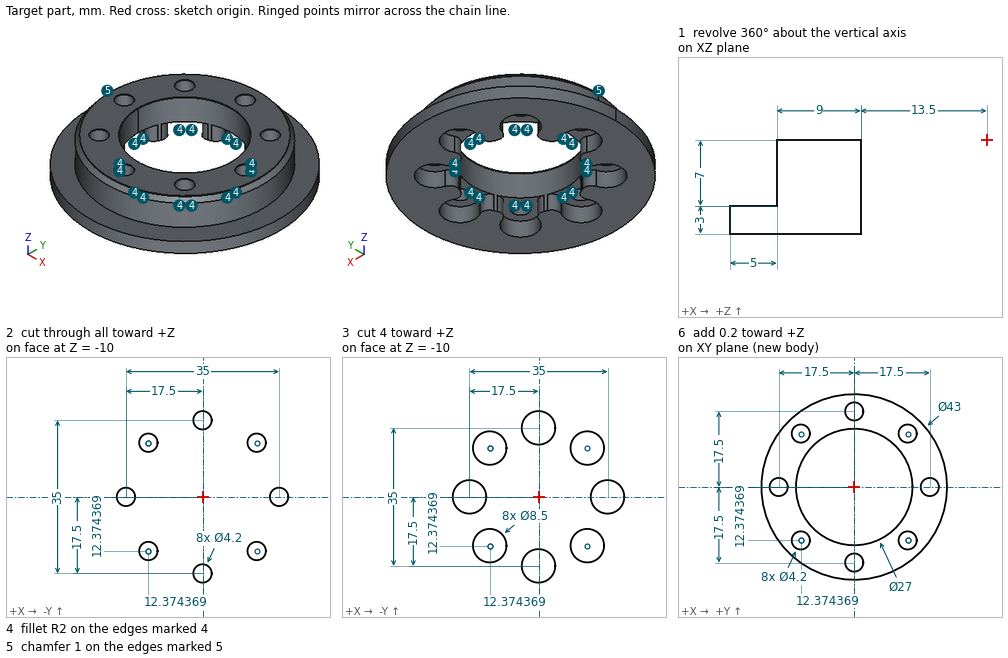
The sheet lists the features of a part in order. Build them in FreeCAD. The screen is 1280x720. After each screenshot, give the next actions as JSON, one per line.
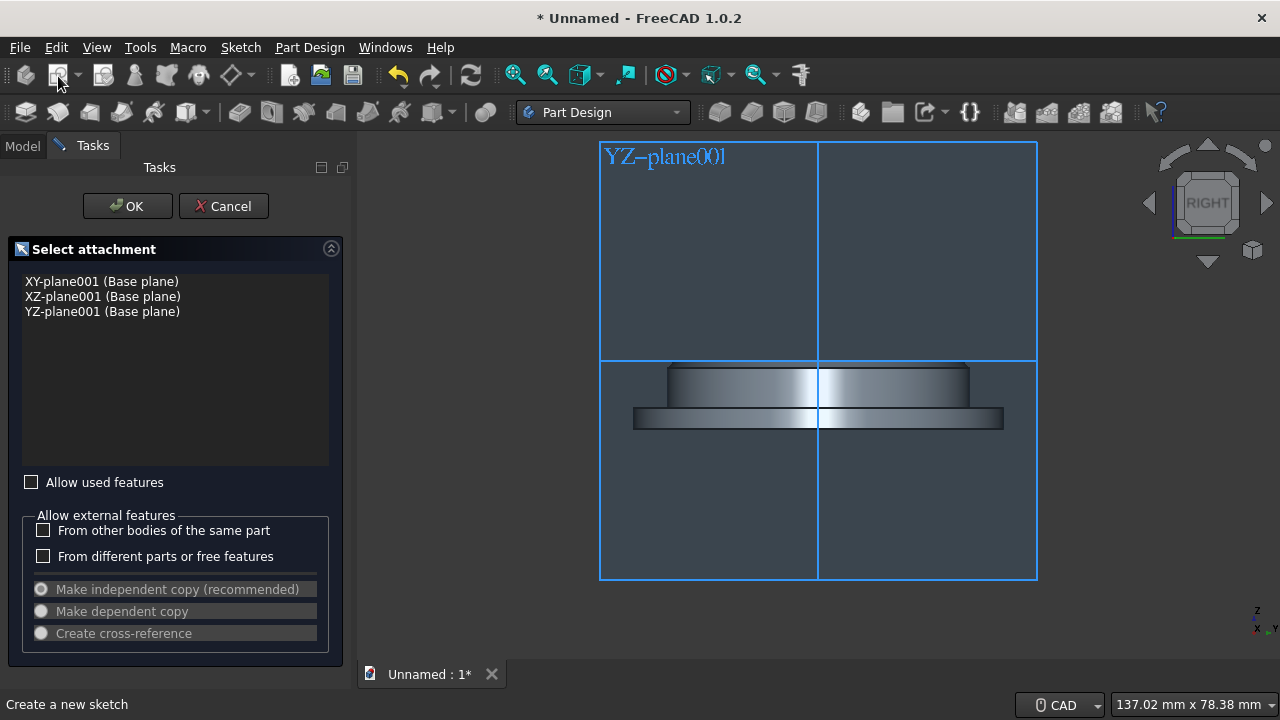
{"action": "left_click", "coordinate": [82, 282]}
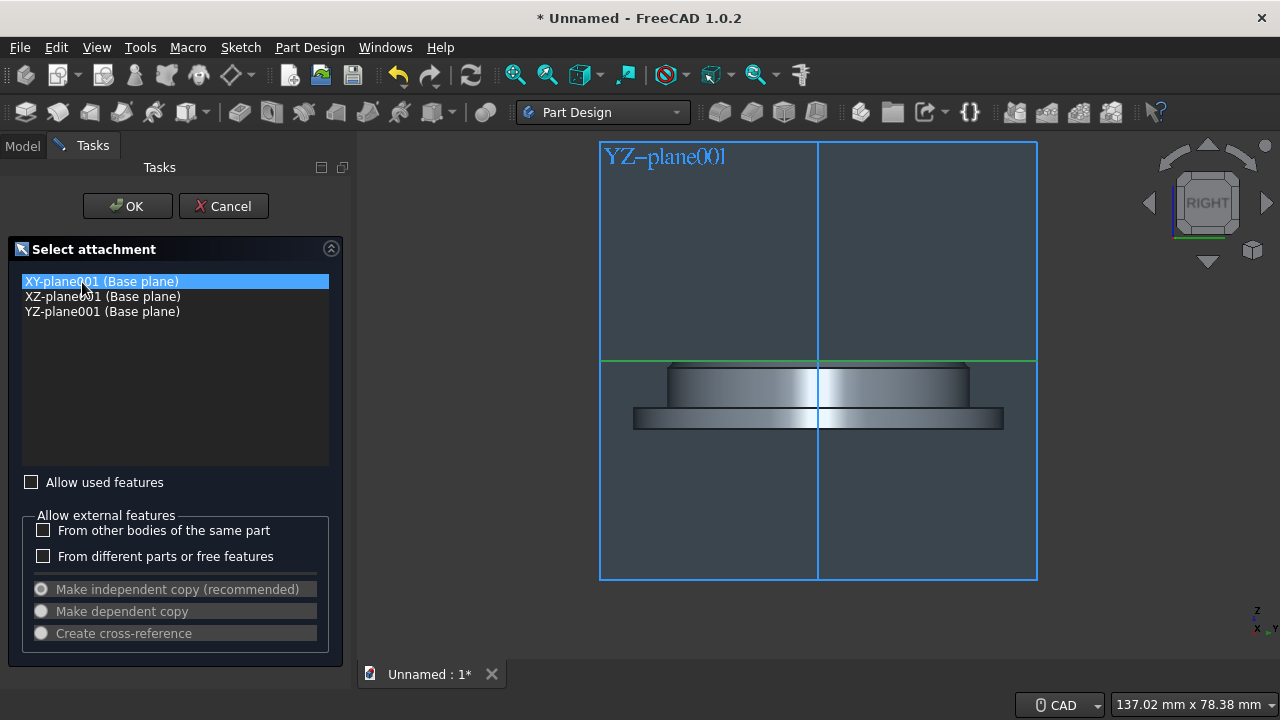
{"action": "left_click", "coordinate": [128, 206]}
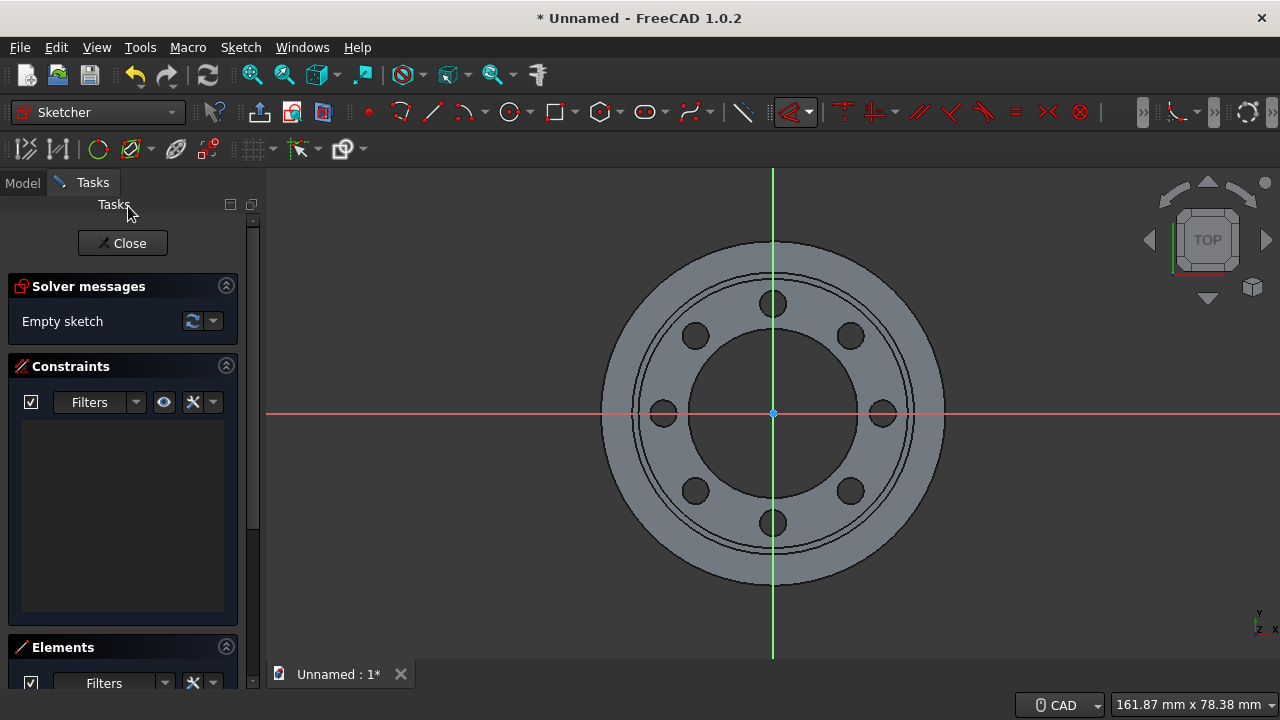
{"action": "left_click", "coordinate": [510, 112]}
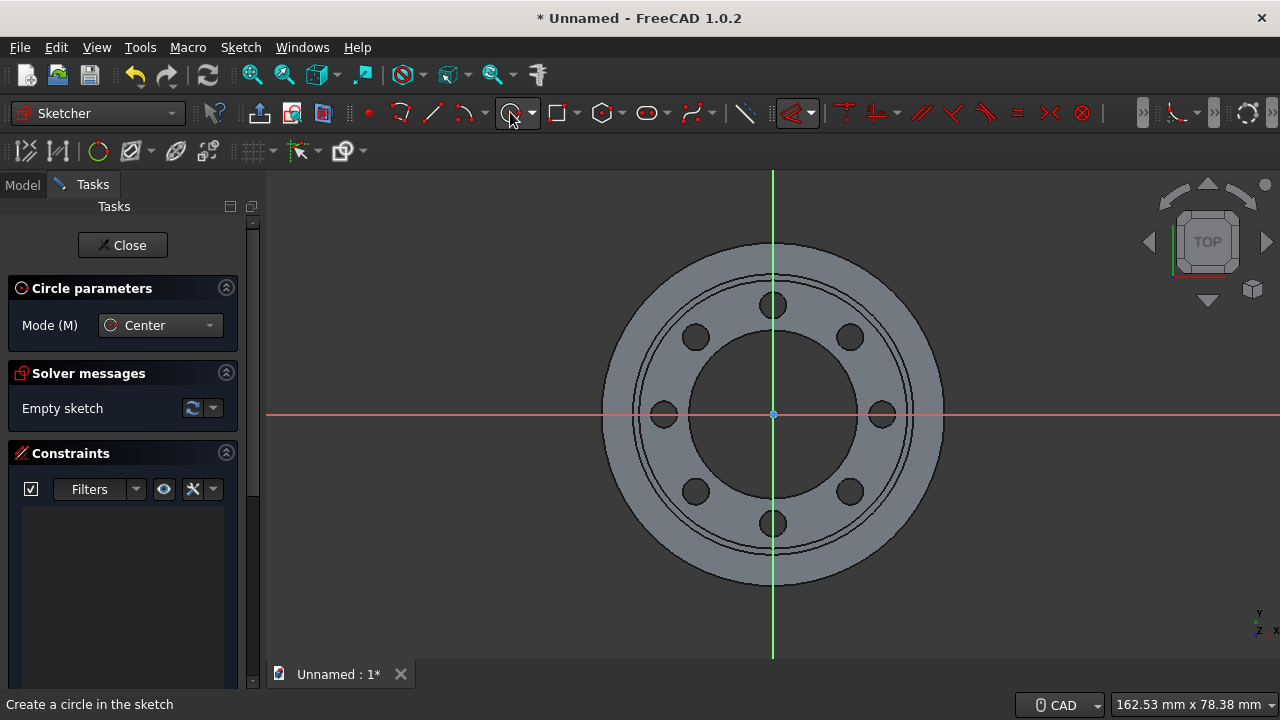
{"action": "left_click", "coordinate": [773, 415]}
{"action": "mouse_move", "coordinate": [868, 320]}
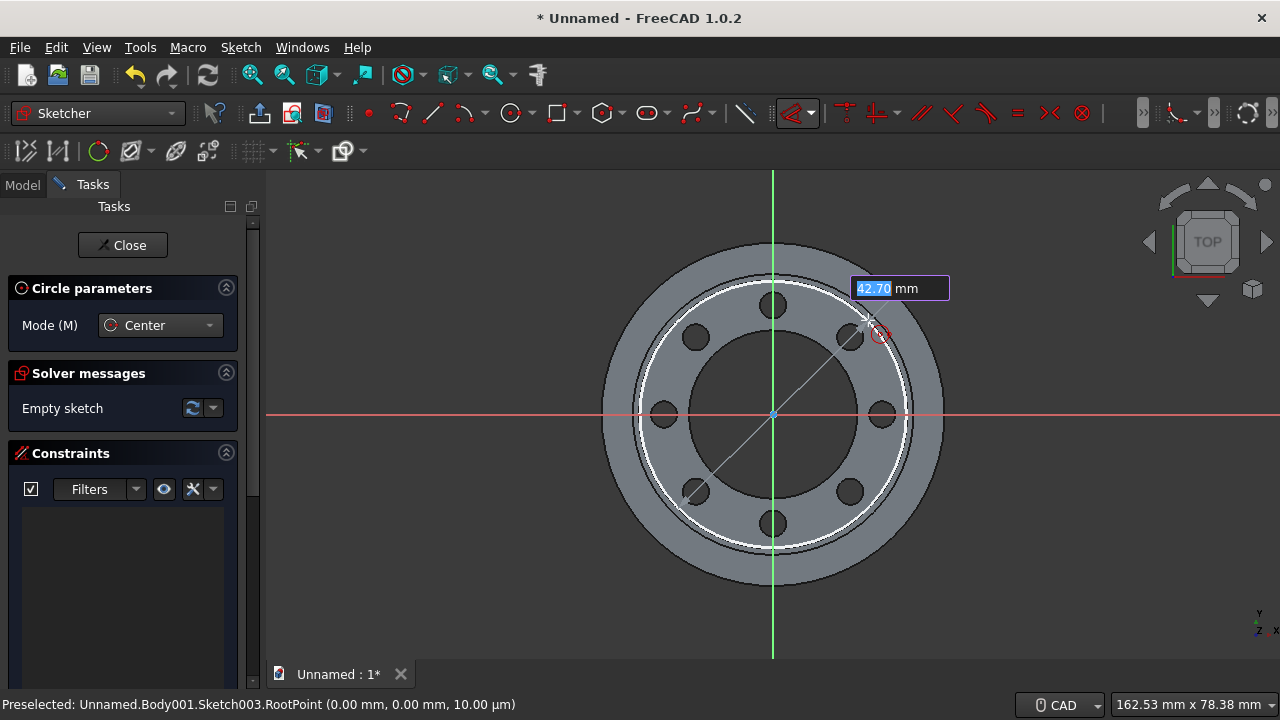
{"action": "type", "text": "43"}
{"action": "key", "text": "Return"}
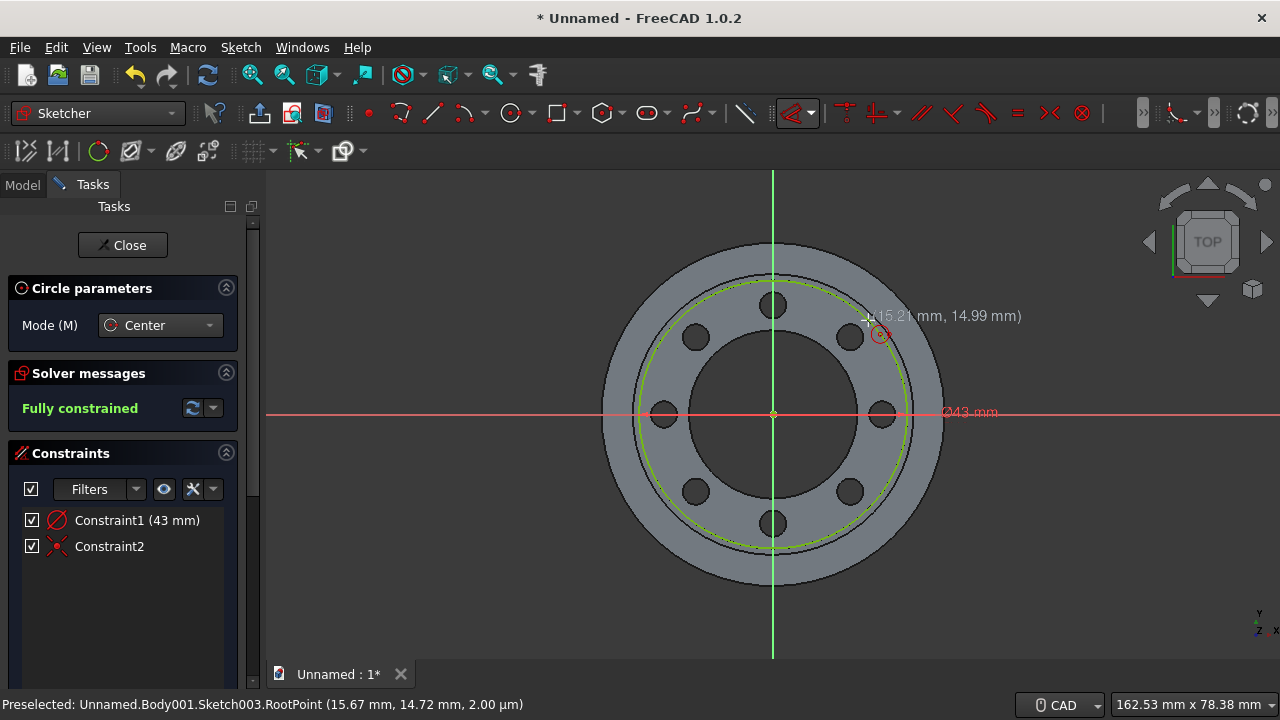
{"action": "scroll", "coordinate": [696, 492], "scroll_direction": "up", "scroll_amount": 3}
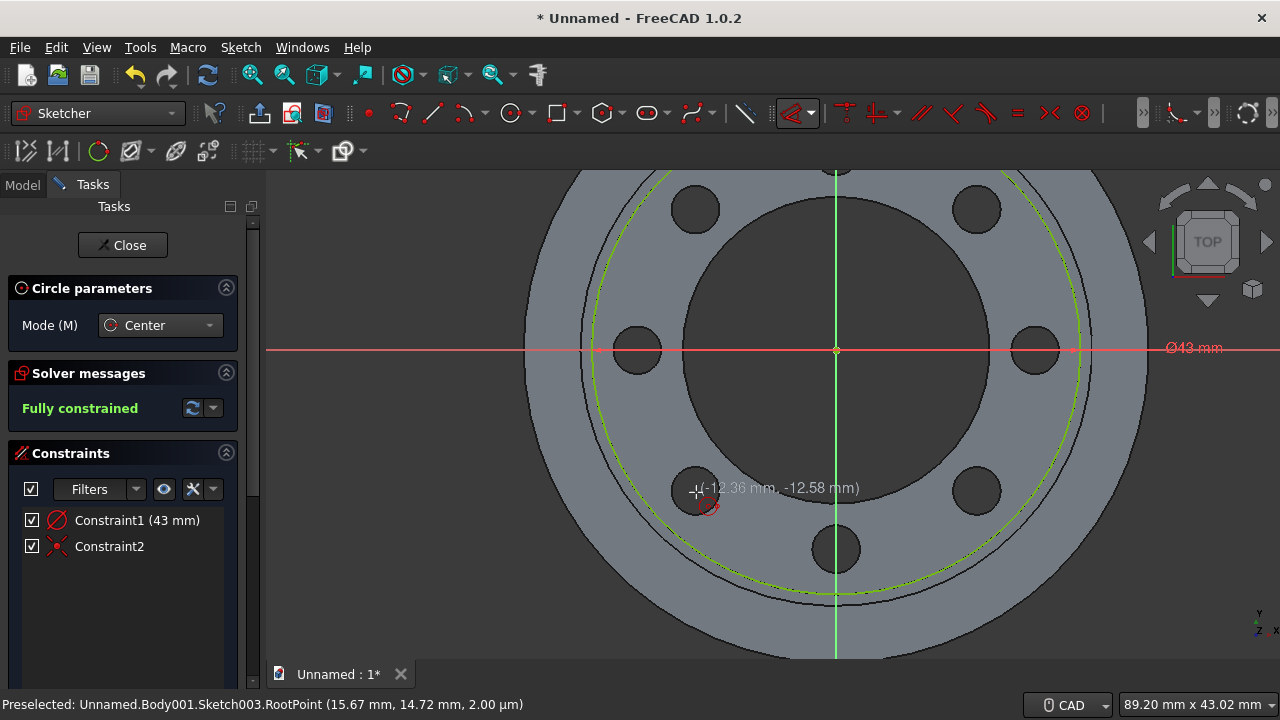
{"action": "left_click", "coordinate": [696, 491]}
{"action": "mouse_move", "coordinate": [712, 474]}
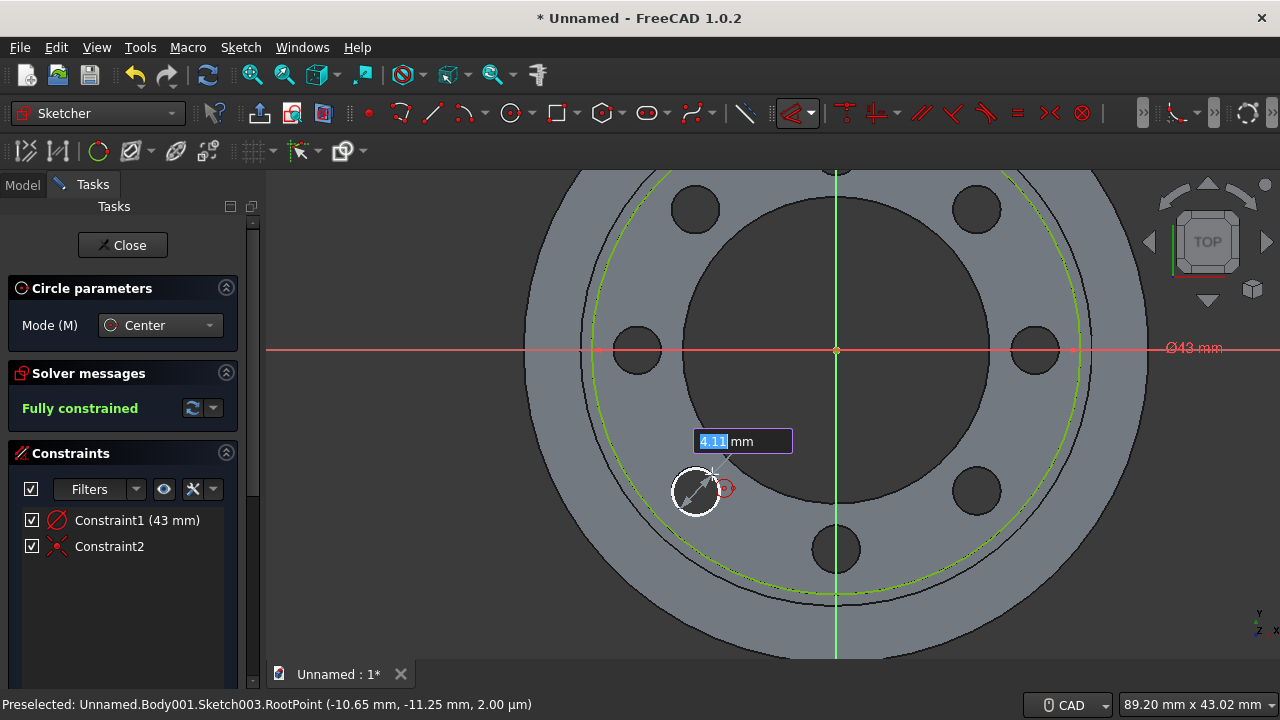
{"action": "type", "text": "4.2"}
{"action": "key", "text": "Return"}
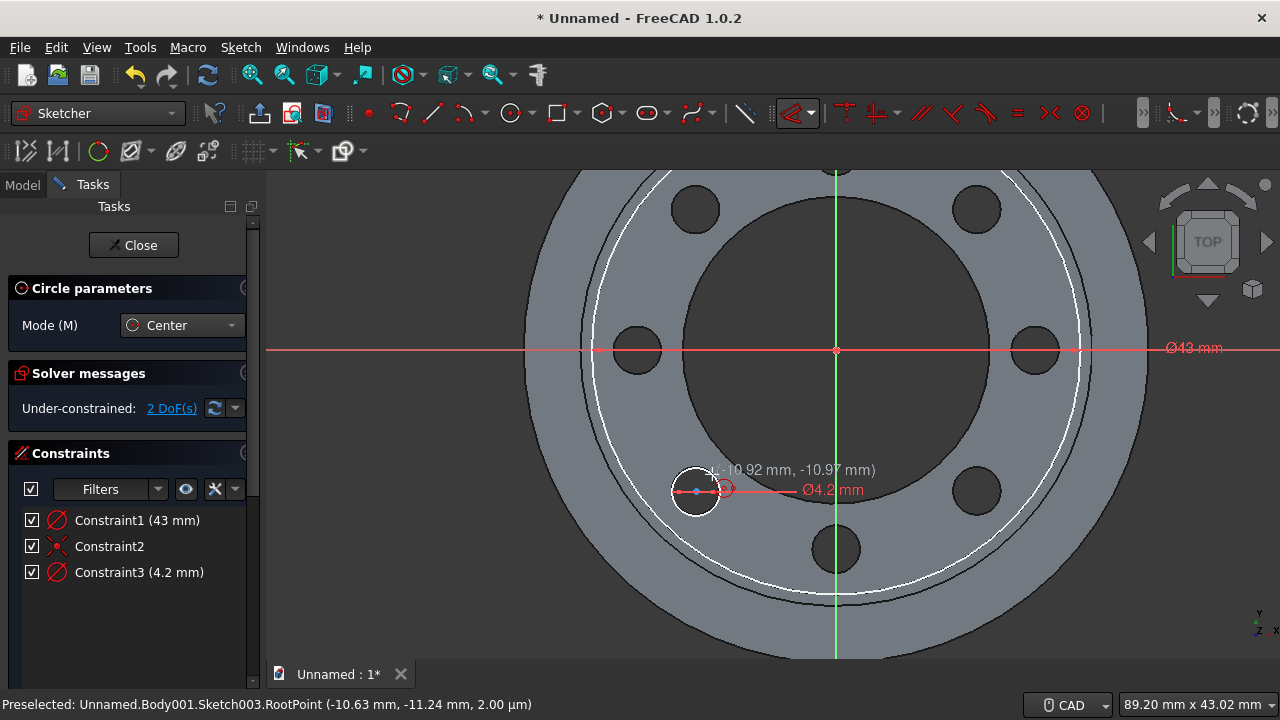
{"action": "left_click", "coordinate": [836, 549]}
{"action": "mouse_move", "coordinate": [853, 532]}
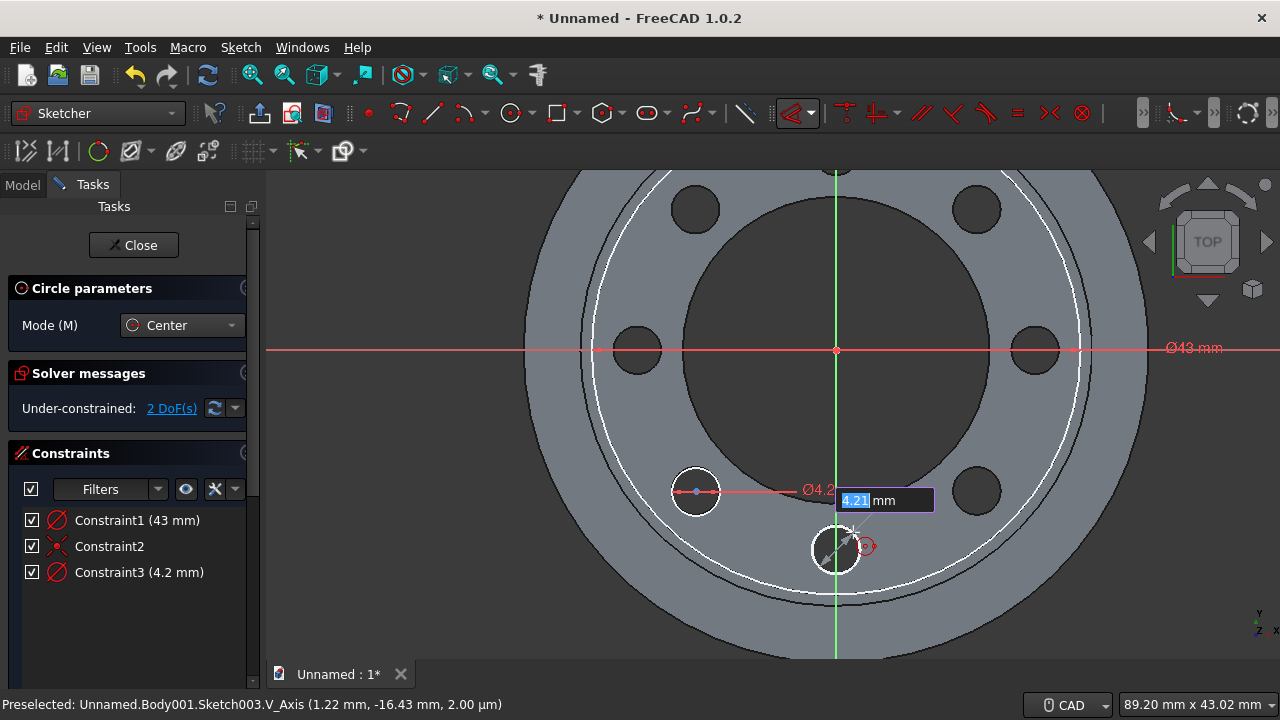
{"action": "type", "text": "4.2"}
{"action": "key", "text": "Return"}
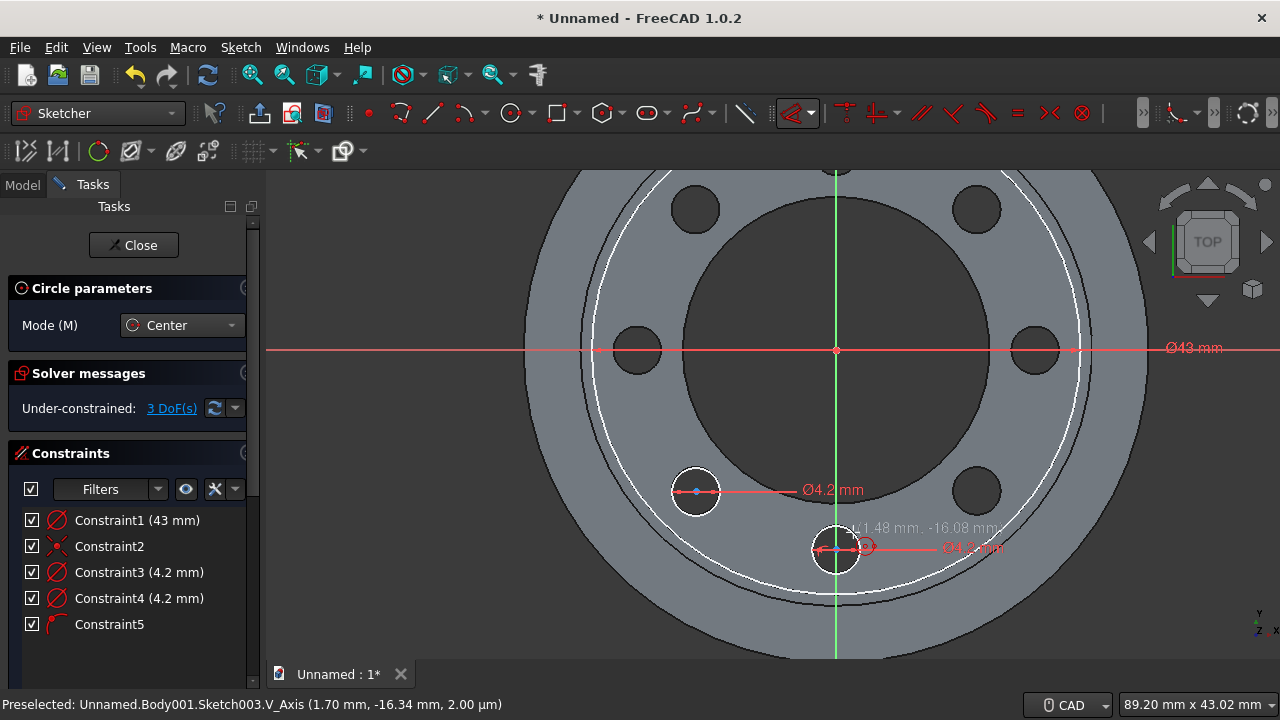
{"action": "left_click", "coordinate": [977, 491]}
{"action": "mouse_move", "coordinate": [994, 474]}